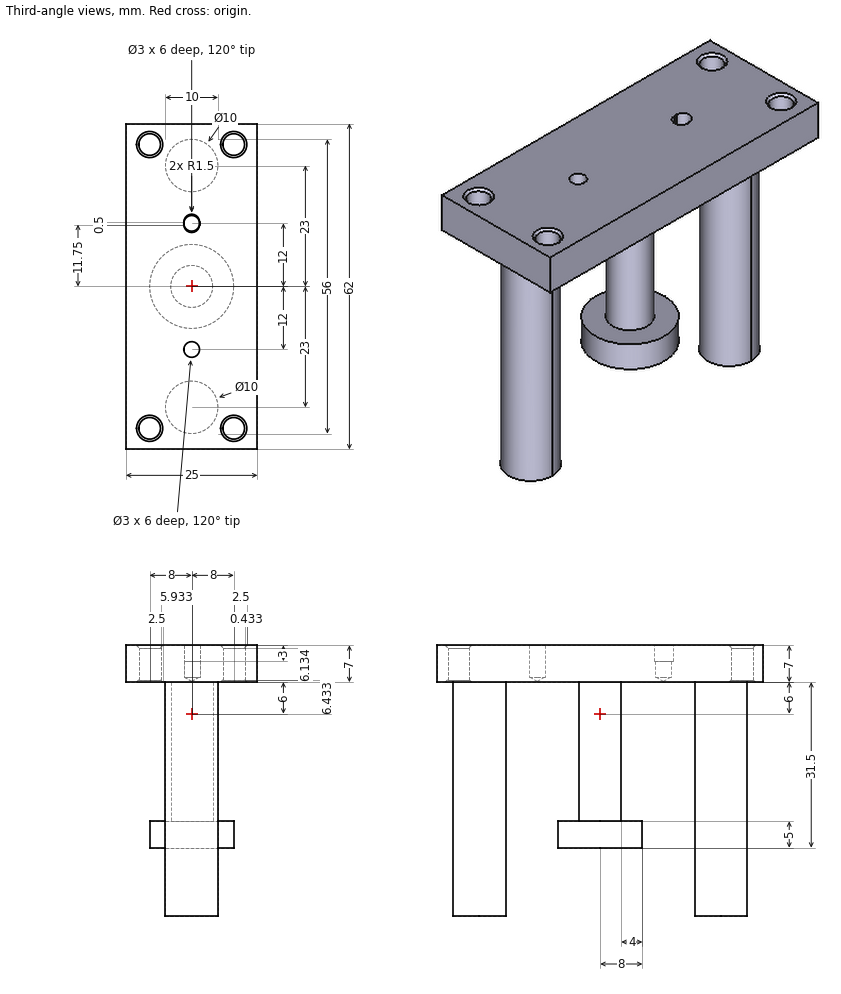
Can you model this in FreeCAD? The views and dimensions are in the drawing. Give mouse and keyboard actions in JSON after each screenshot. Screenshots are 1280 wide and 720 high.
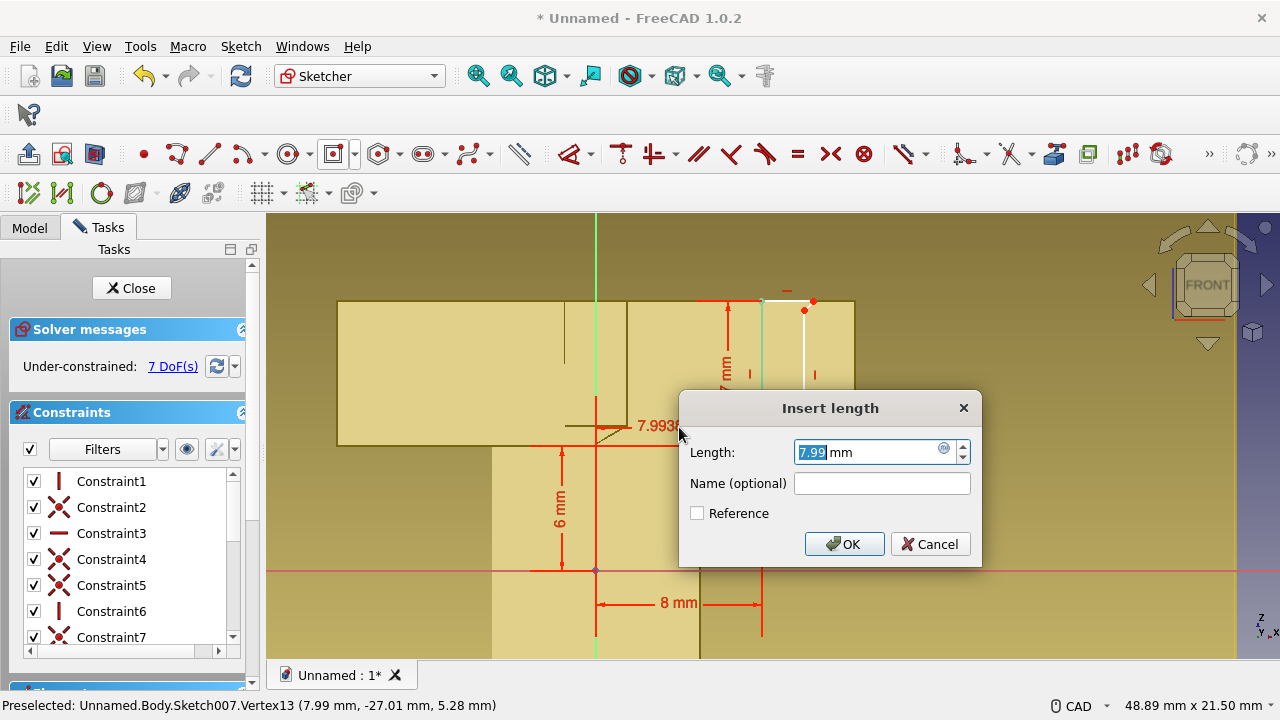
{"action": "type", "text": "8"}
{"action": "key", "text": "Return"}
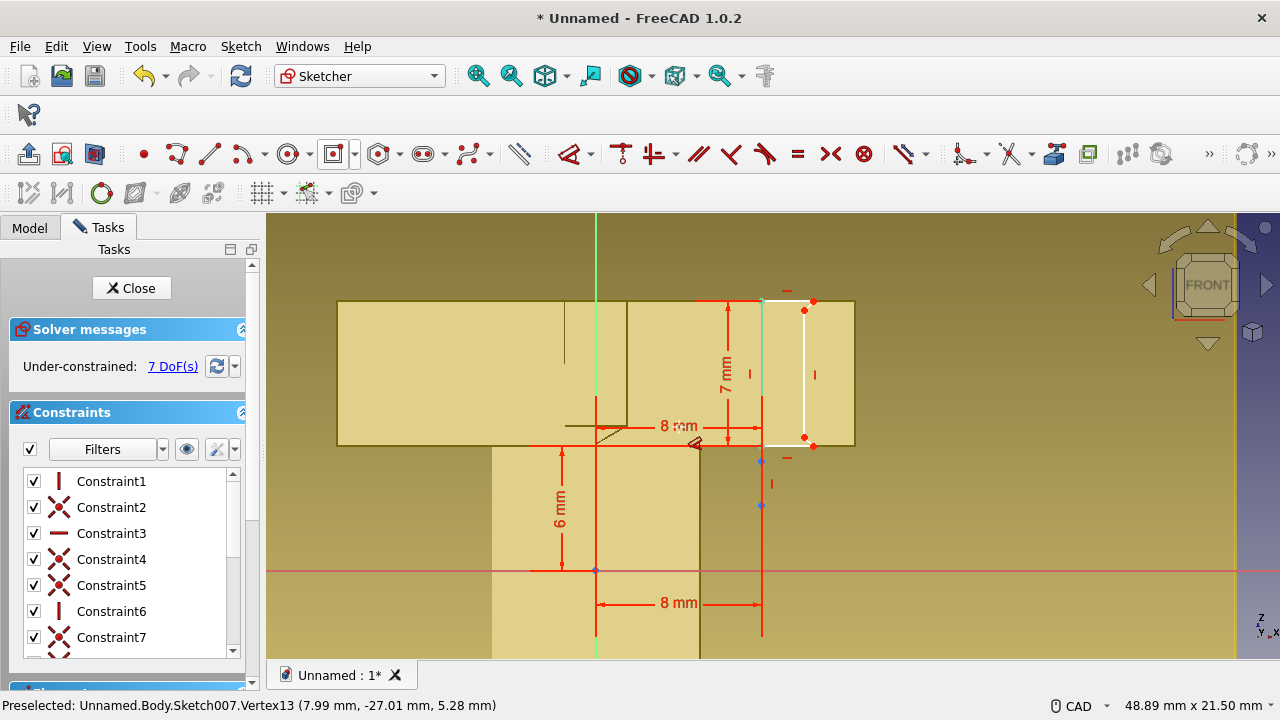
{"action": "left_click", "coordinate": [777, 301]}
{"action": "left_click", "coordinate": [788, 267]}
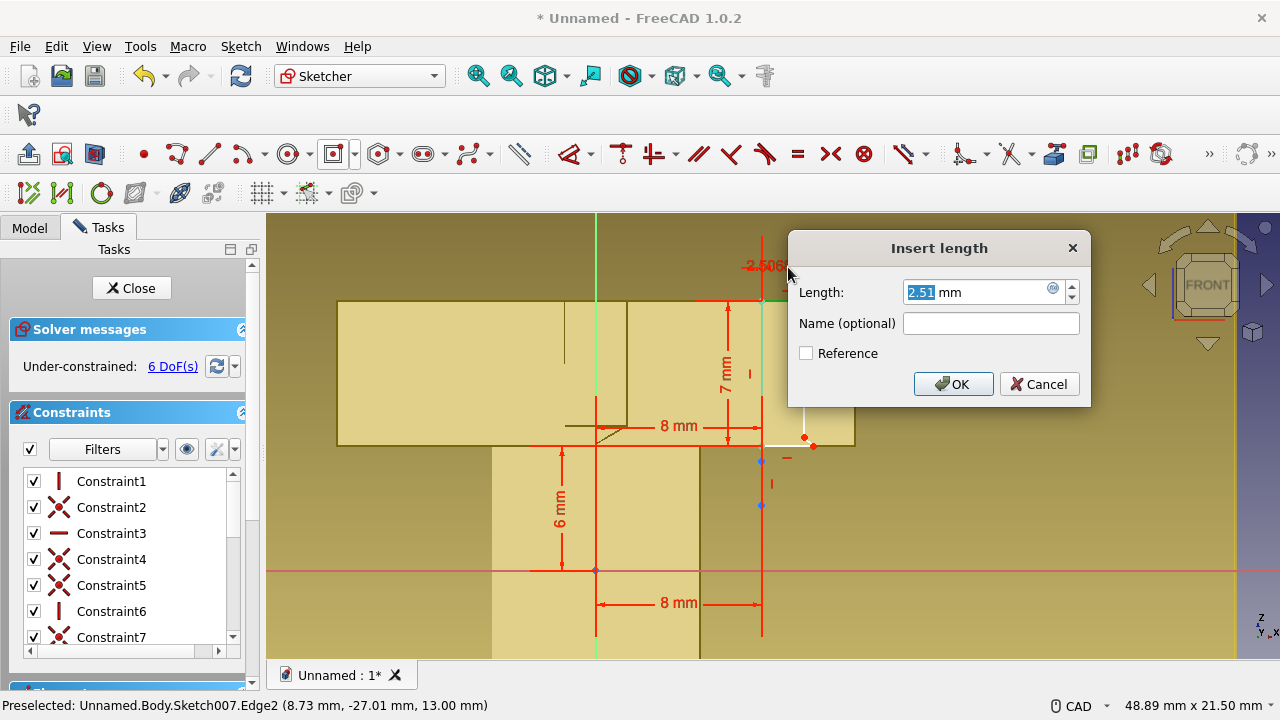
{"action": "type", "text": "2.5"}
{"action": "key", "text": "Return"}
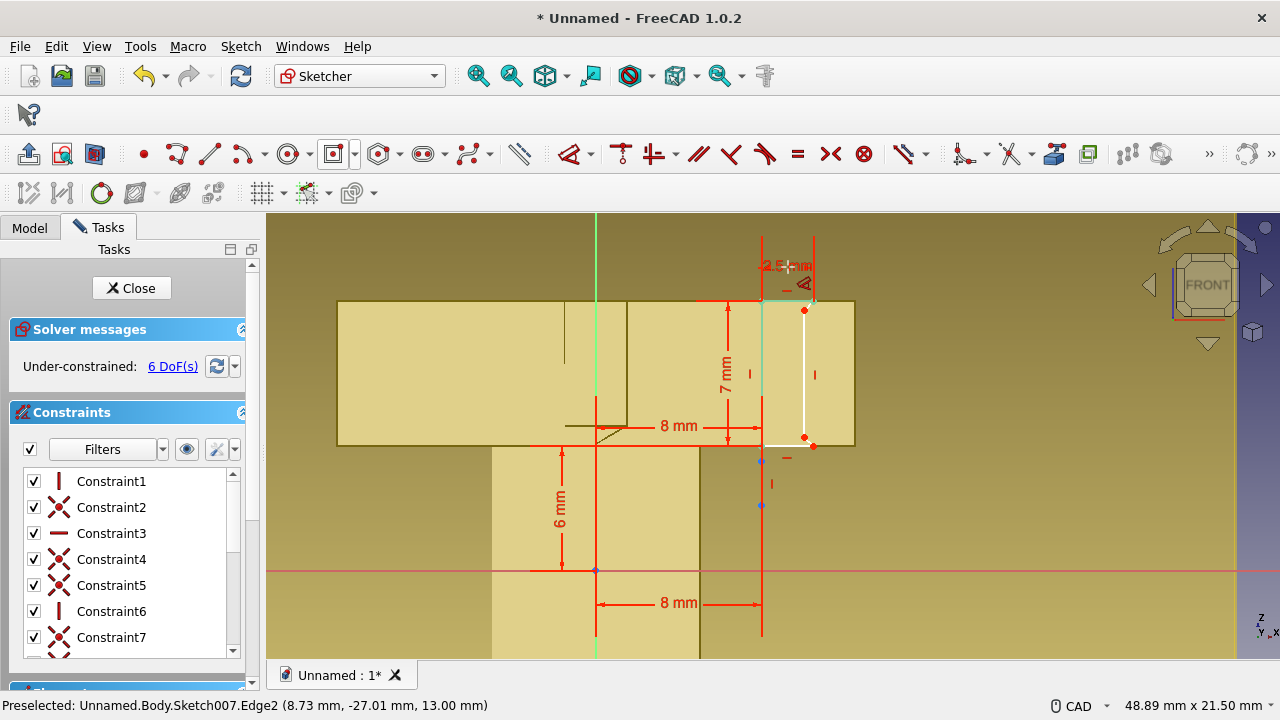
{"action": "scroll", "coordinate": [798, 446], "scroll_direction": "up", "scroll_amount": 2}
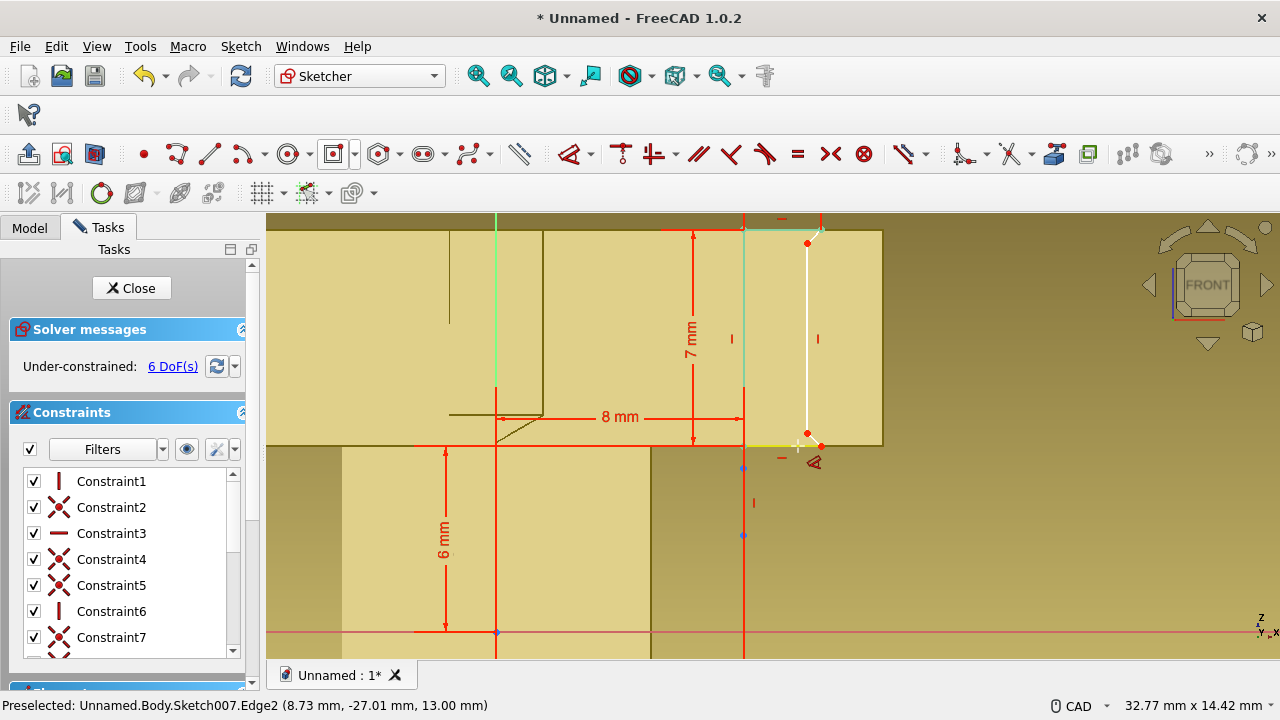
{"action": "left_click", "coordinate": [798, 446]}
{"action": "left_click", "coordinate": [783, 480]}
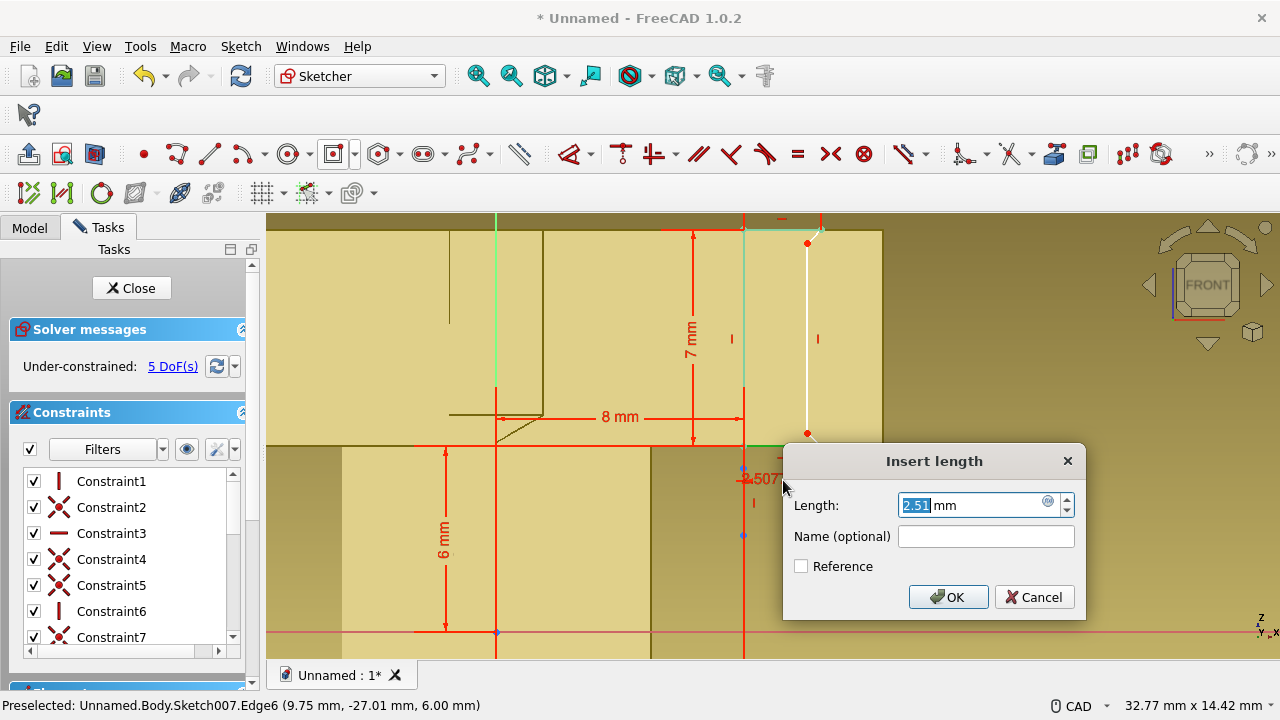
{"action": "type", "text": "2.5"}
{"action": "key", "text": "Return"}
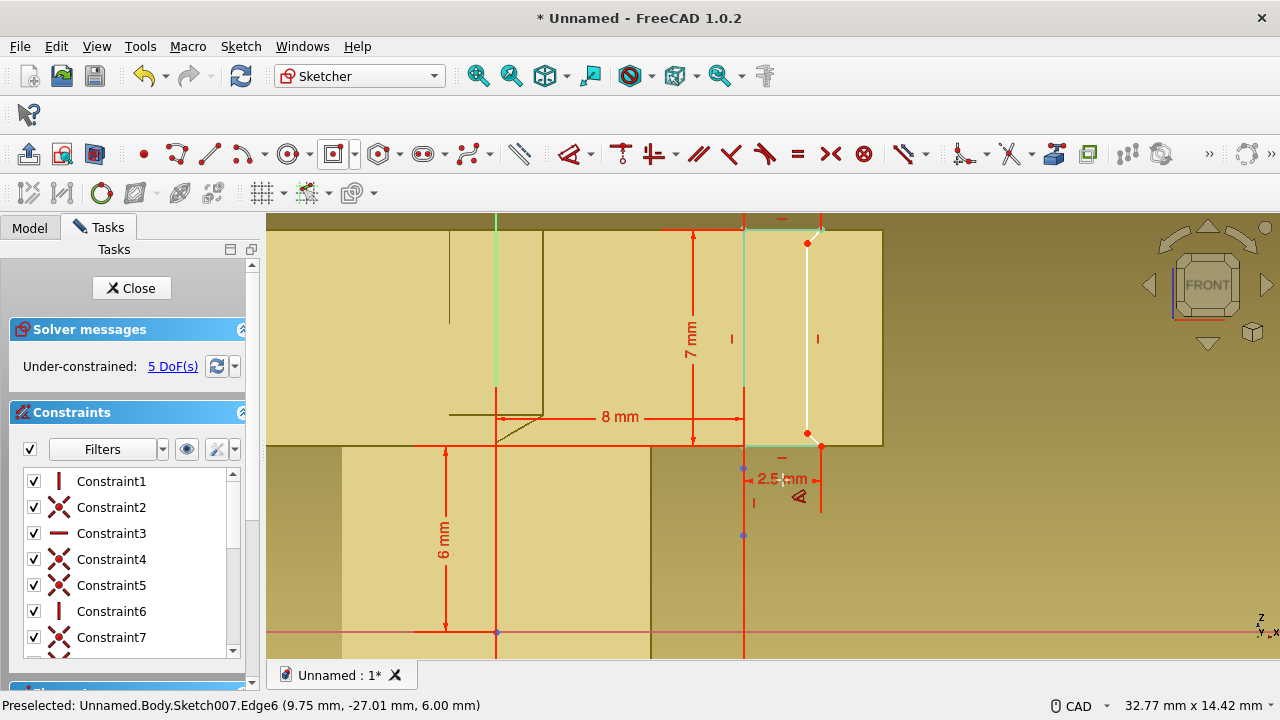
{"action": "left_click", "coordinate": [807, 301]}
{"action": "left_click", "coordinate": [841, 339]}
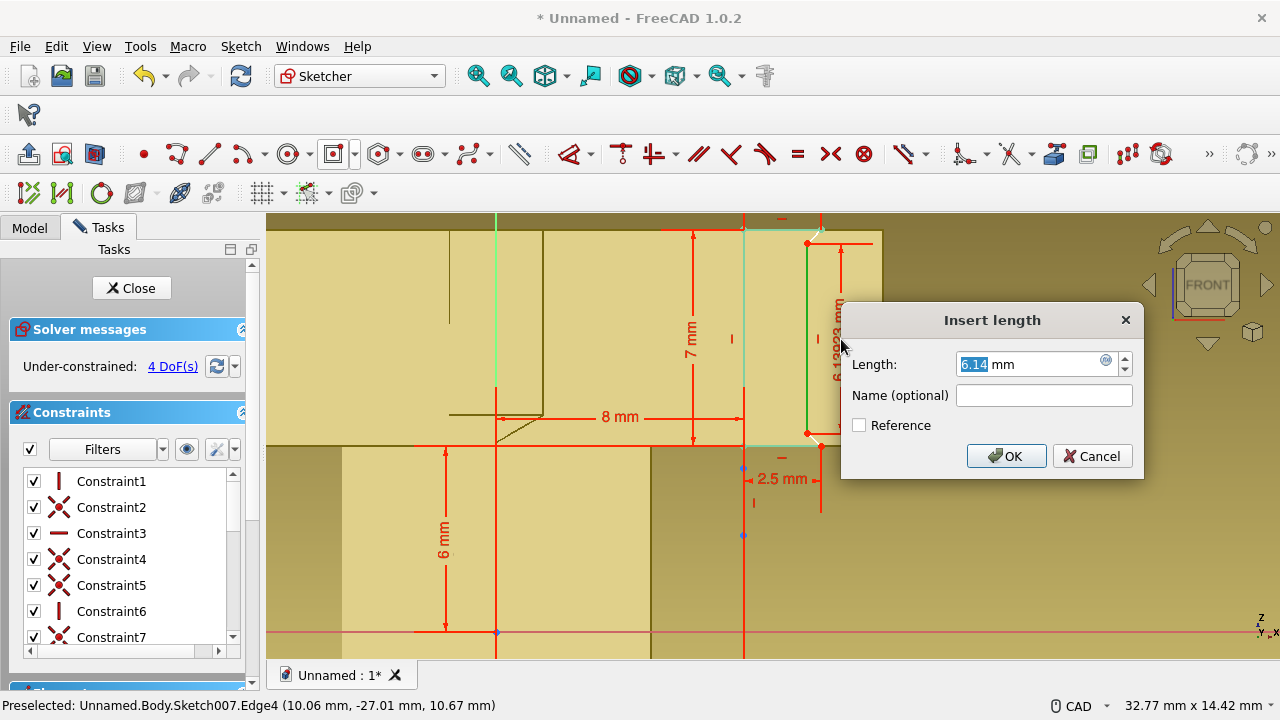
{"action": "type", "text": "6.134"}
{"action": "key", "text": "Return"}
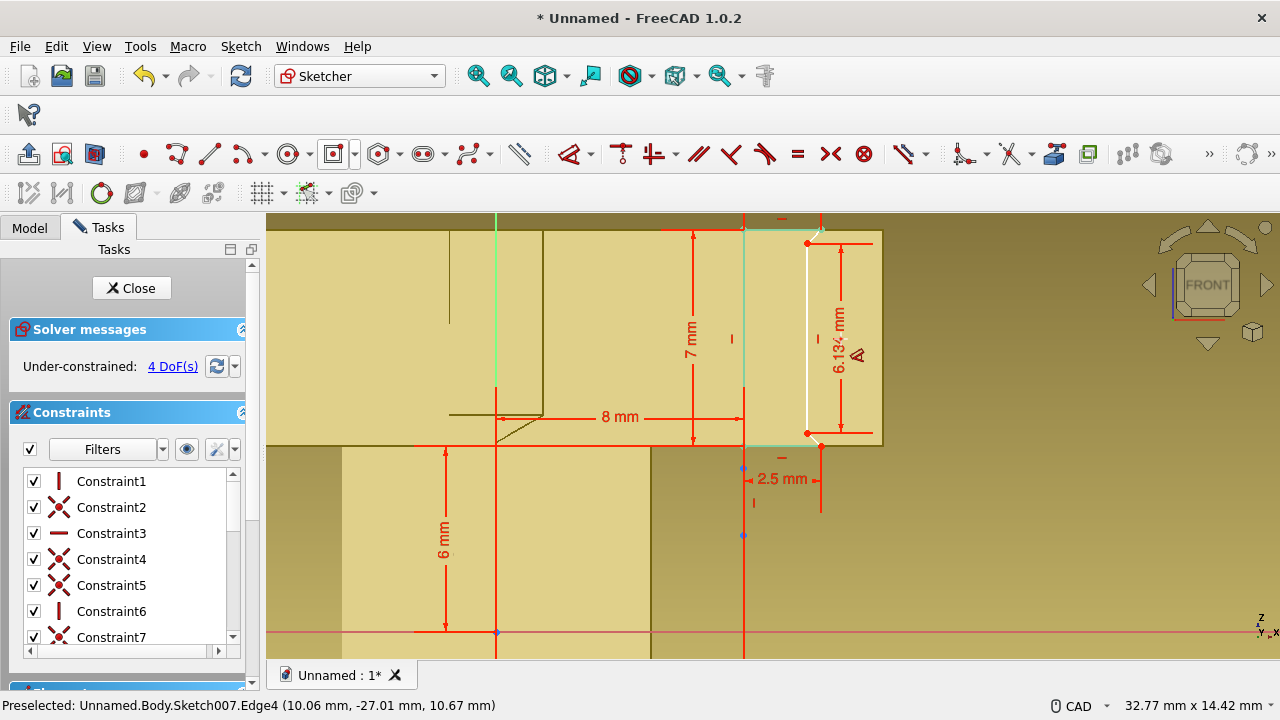
{"action": "left_click", "coordinate": [807, 433]}
{"action": "left_click", "coordinate": [462, 487]}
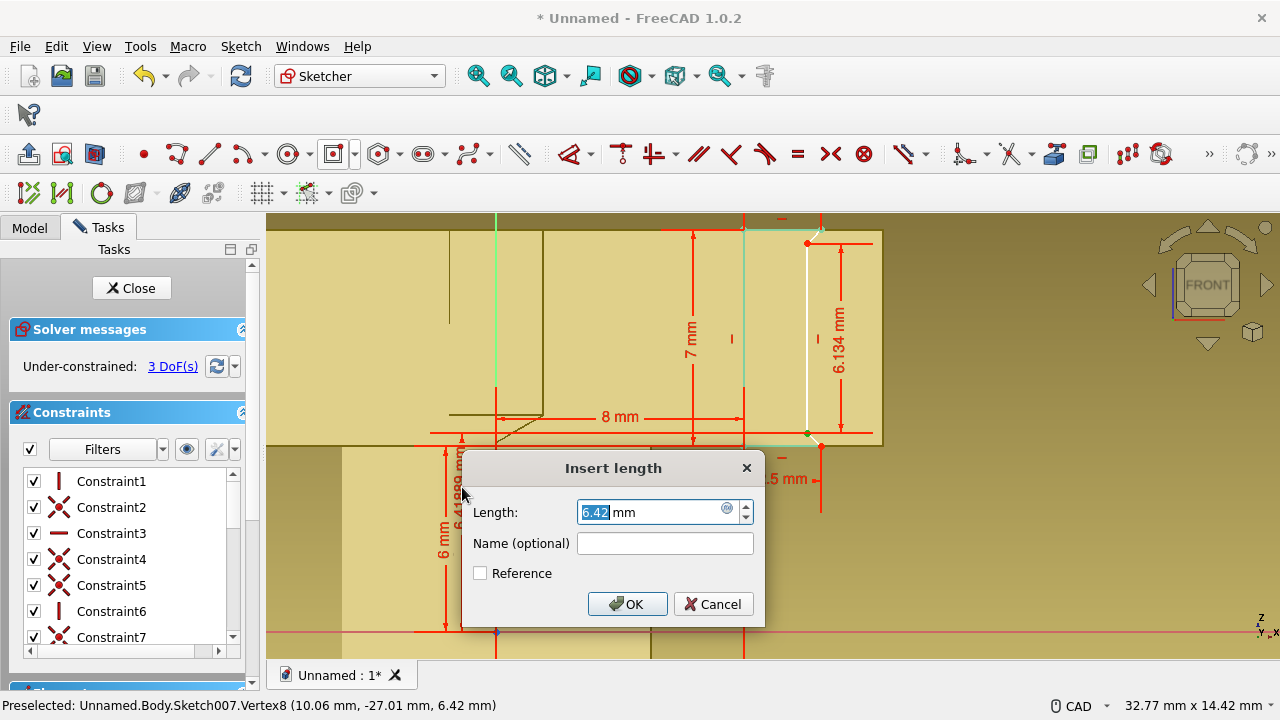
{"action": "type", "text": "6.433"}
{"action": "key", "text": "Return"}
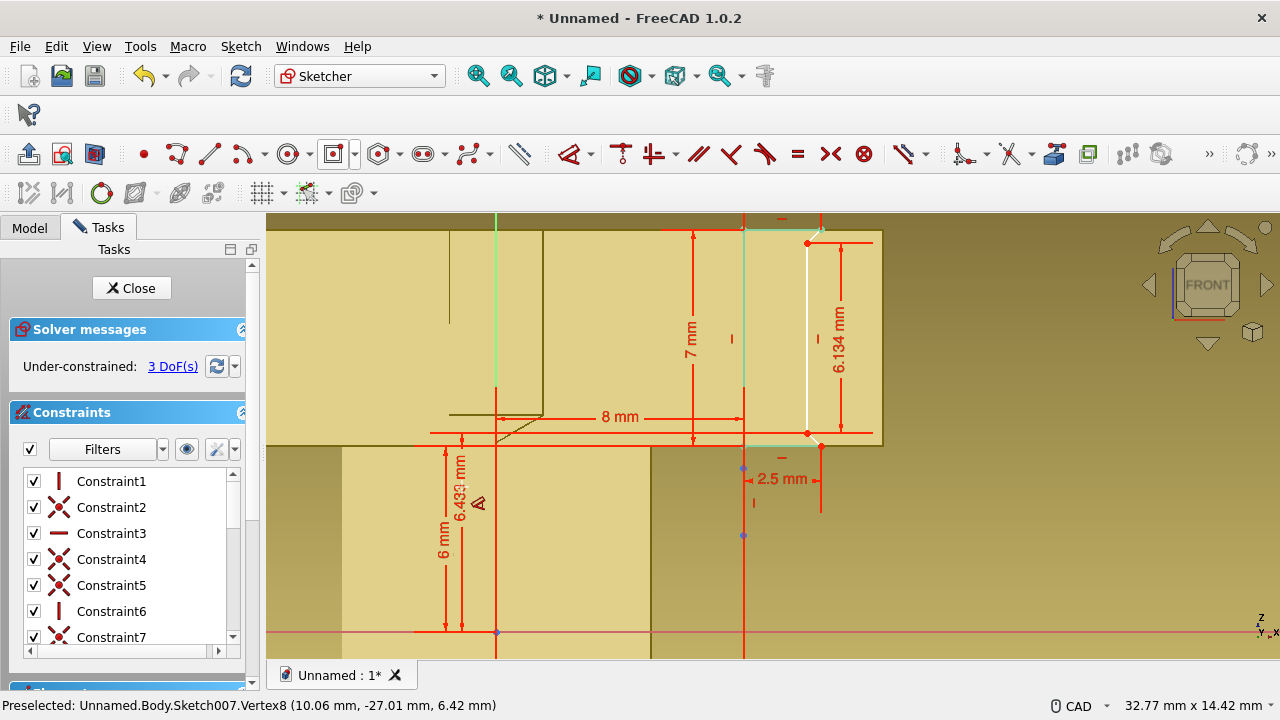
{"action": "scroll", "coordinate": [798, 446], "scroll_direction": "down", "scroll_amount": 2}